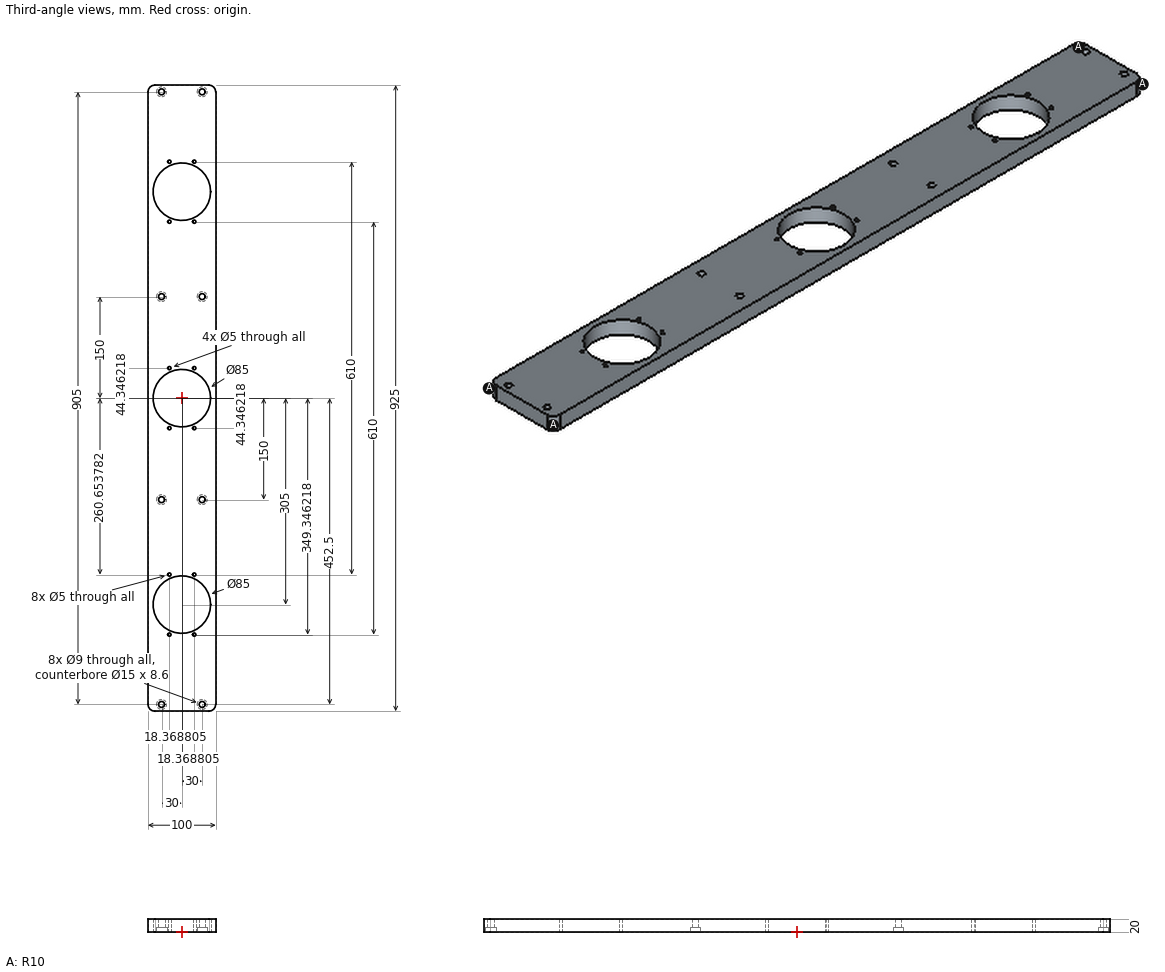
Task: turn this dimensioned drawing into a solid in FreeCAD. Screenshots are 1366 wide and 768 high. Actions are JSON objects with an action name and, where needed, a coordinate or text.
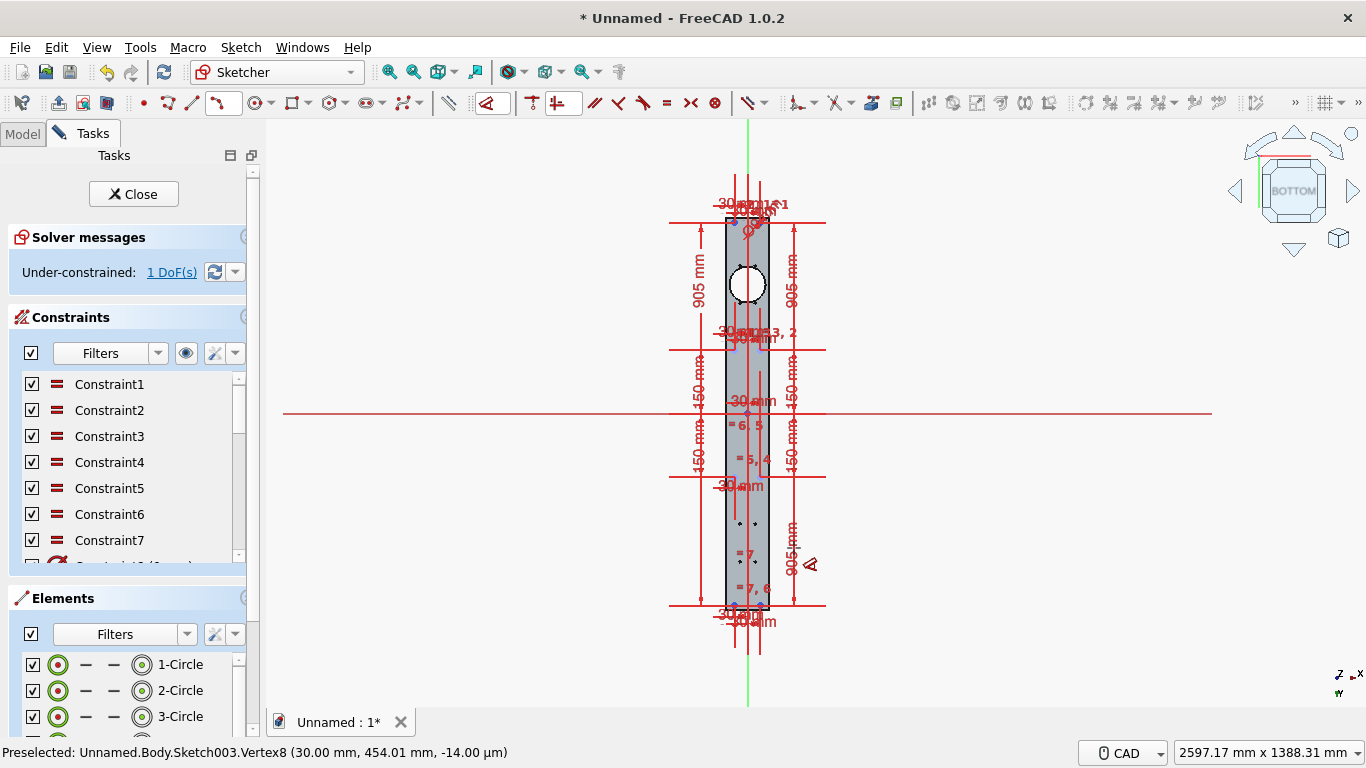
{"action": "left_click", "coordinate": [760, 223]}
{"action": "left_click", "coordinate": [794, 362]}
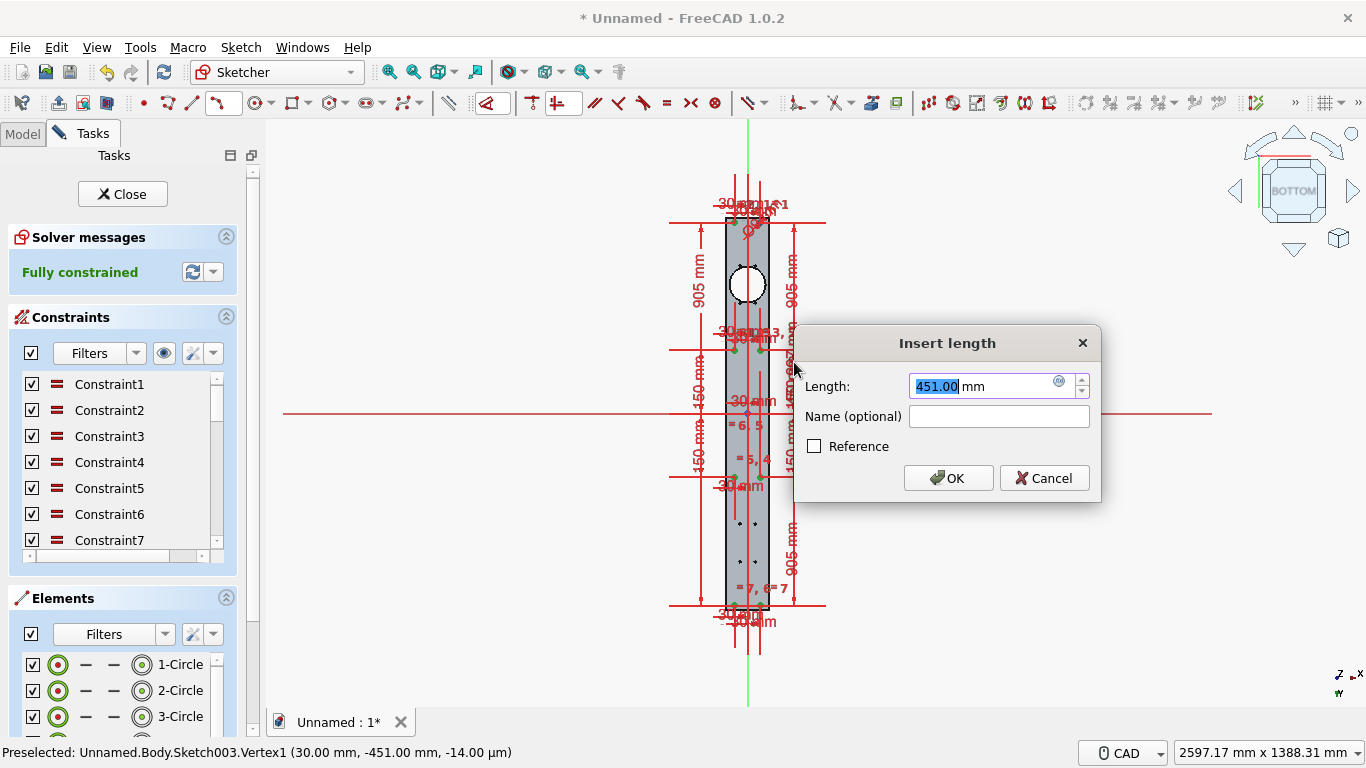
{"action": "type", "text": "452.5"}
{"action": "key", "text": "Return"}
{"action": "key", "text": "Escape"}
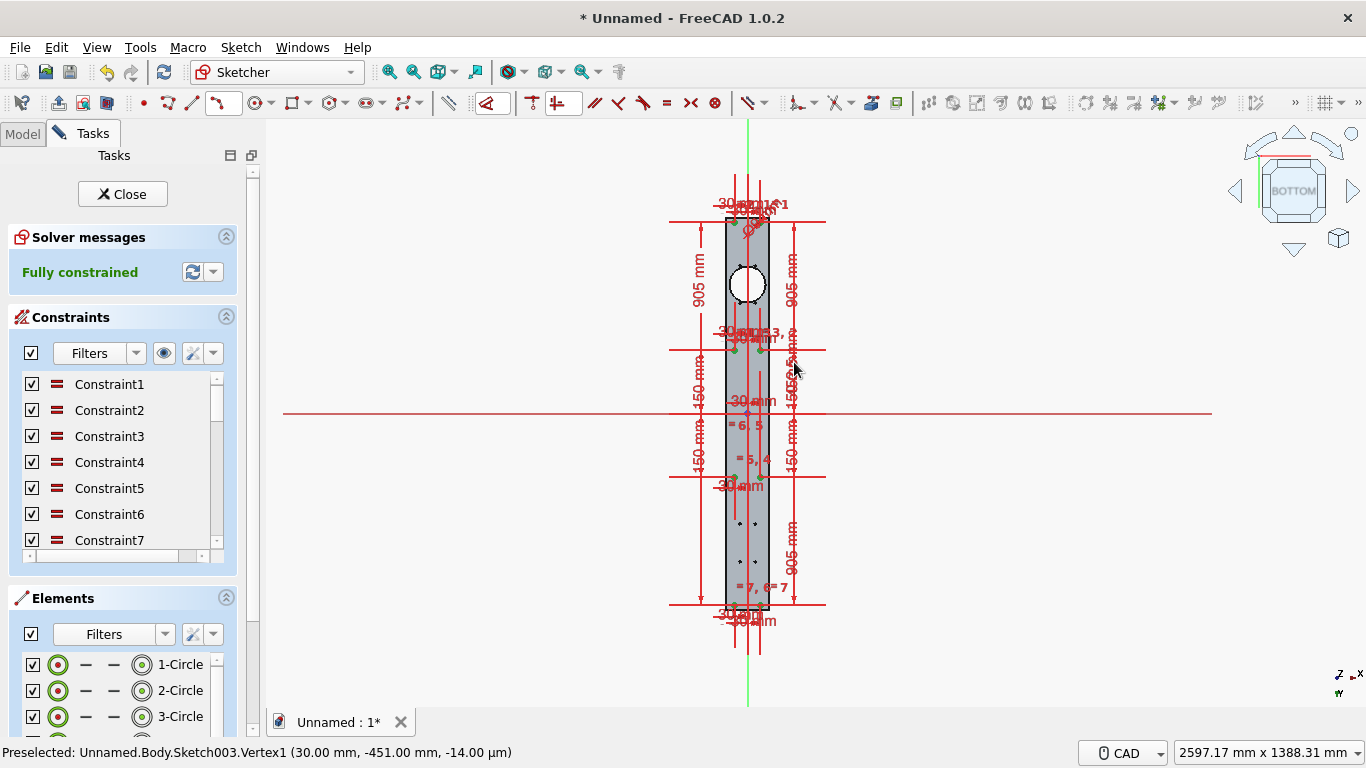
{"action": "left_click", "coordinate": [123, 194]}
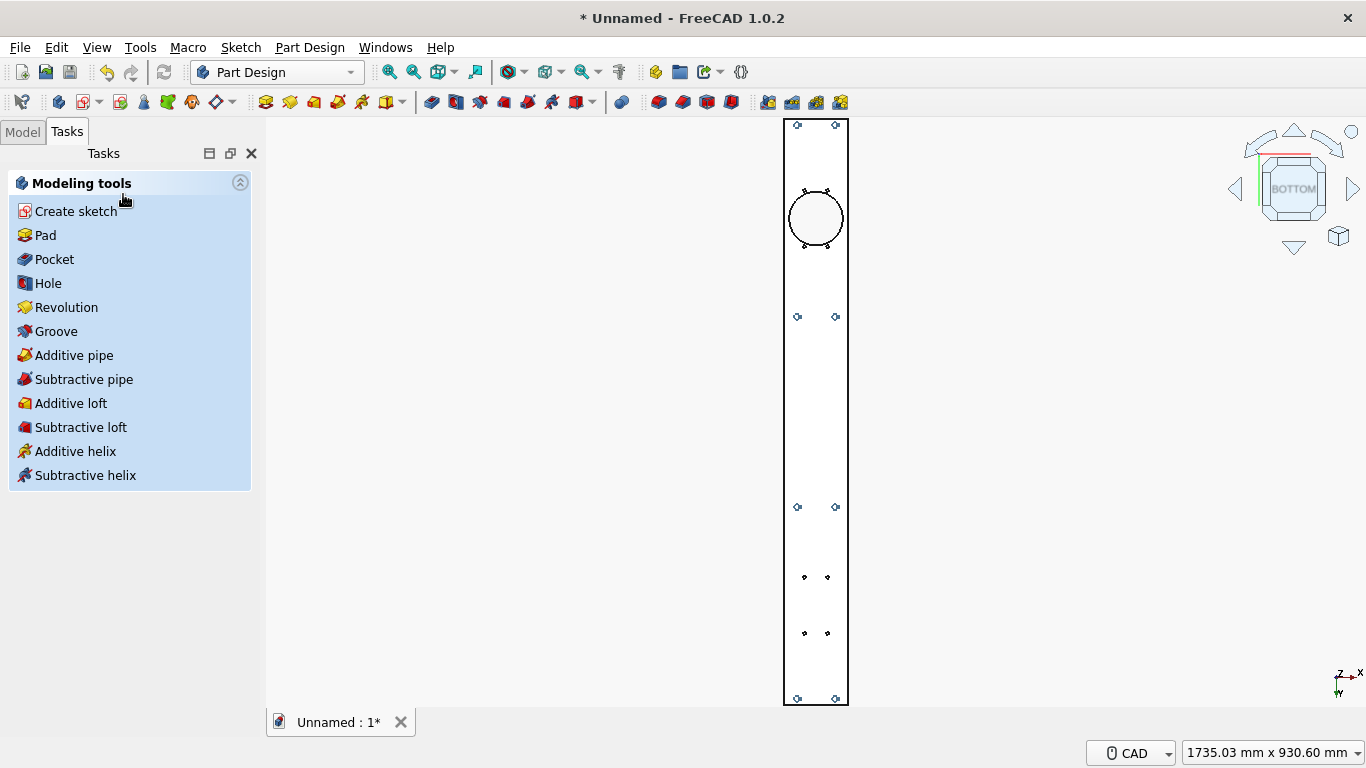
{"action": "left_click", "coordinate": [456, 102]}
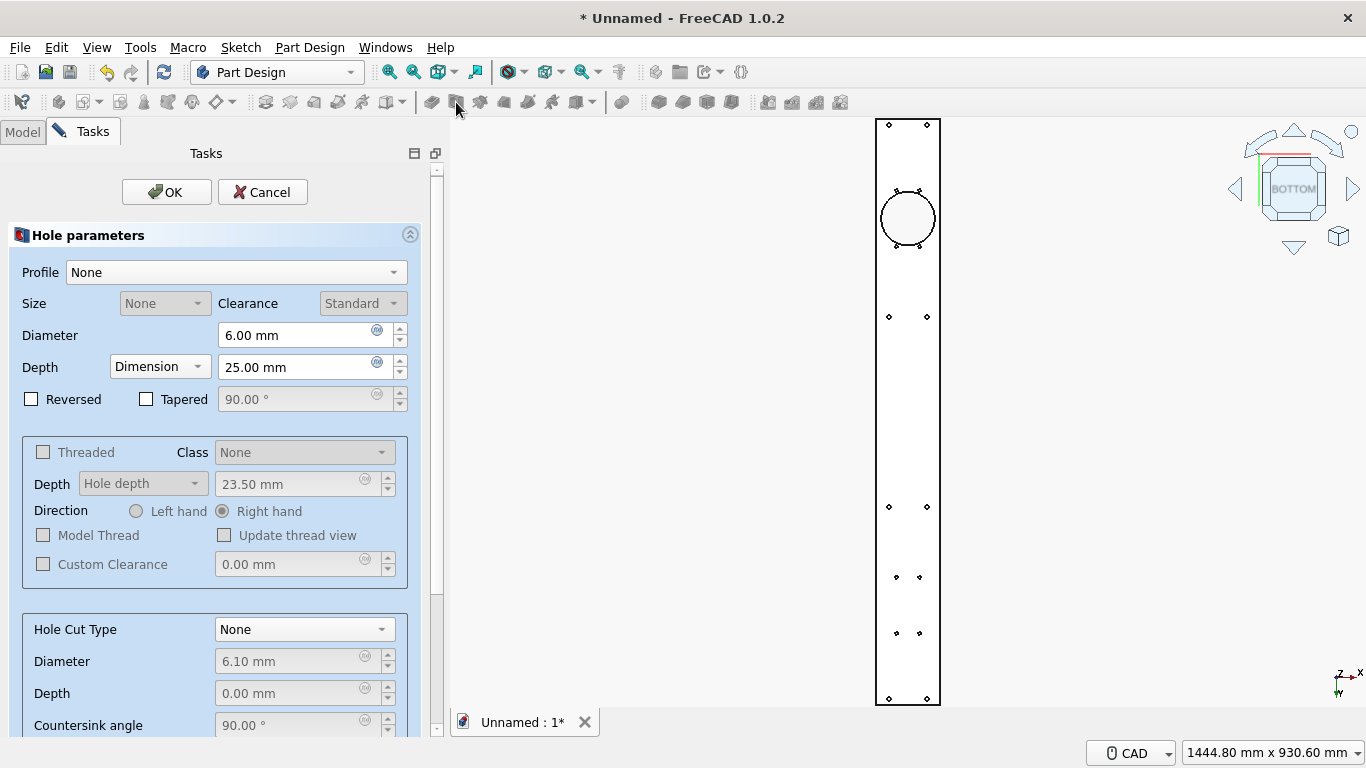
{"action": "triple_click", "coordinate": [305, 335]}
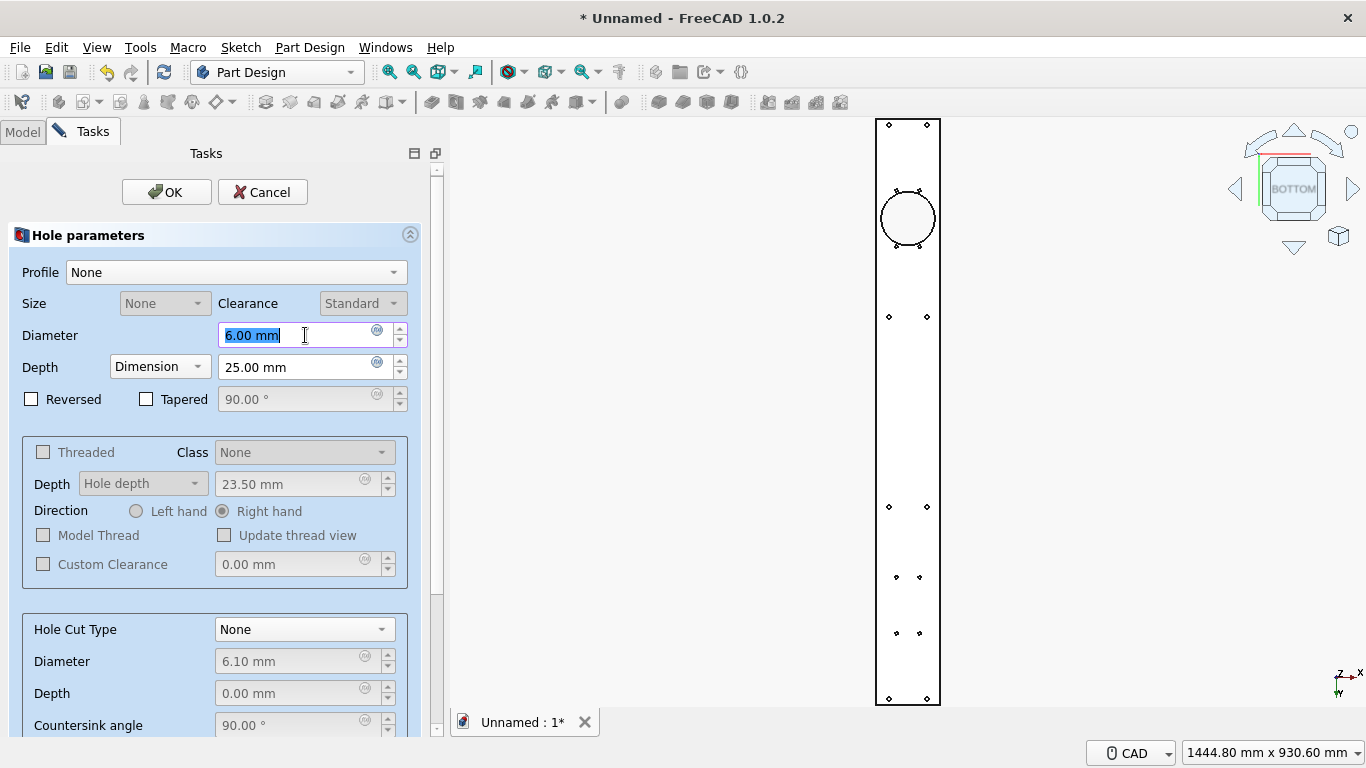
{"action": "type", "text": "9"}
{"action": "key", "text": "Tab"}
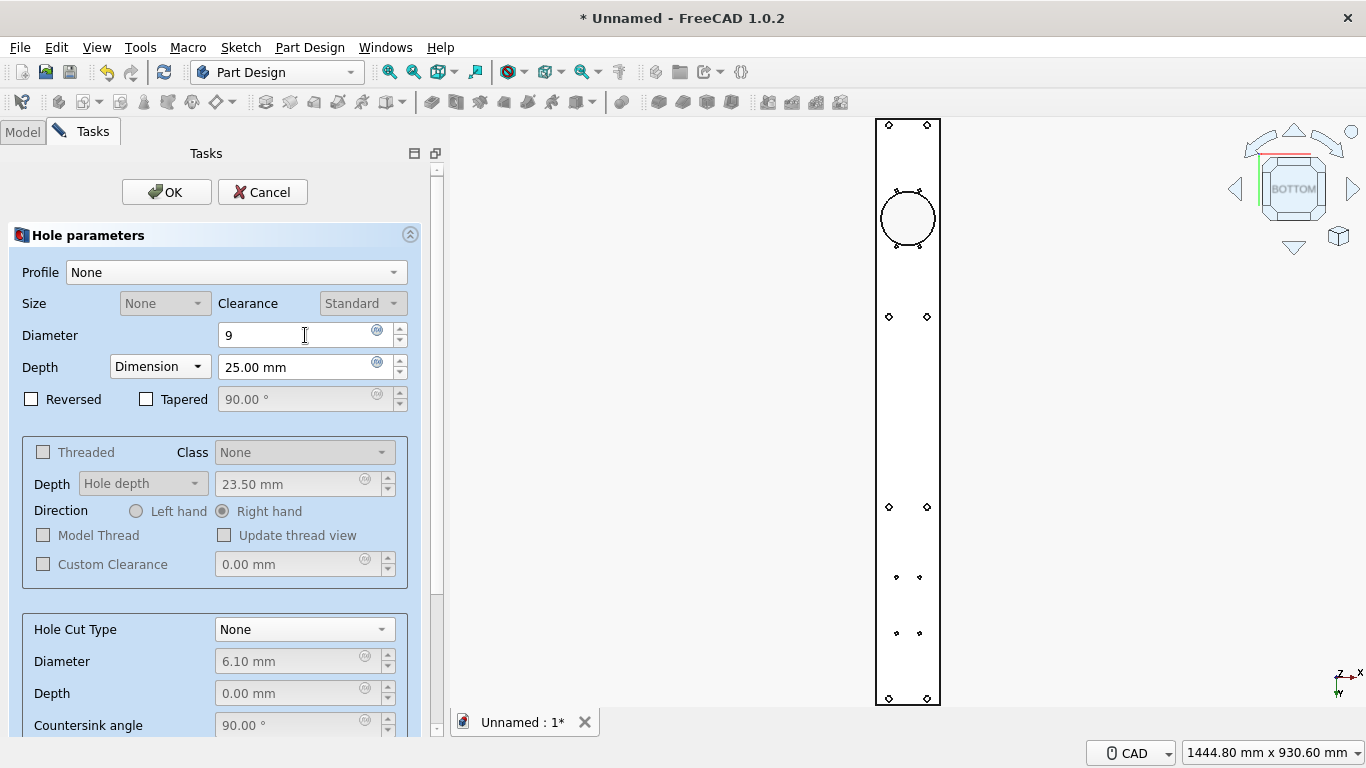
{"action": "left_click", "coordinate": [161, 366]}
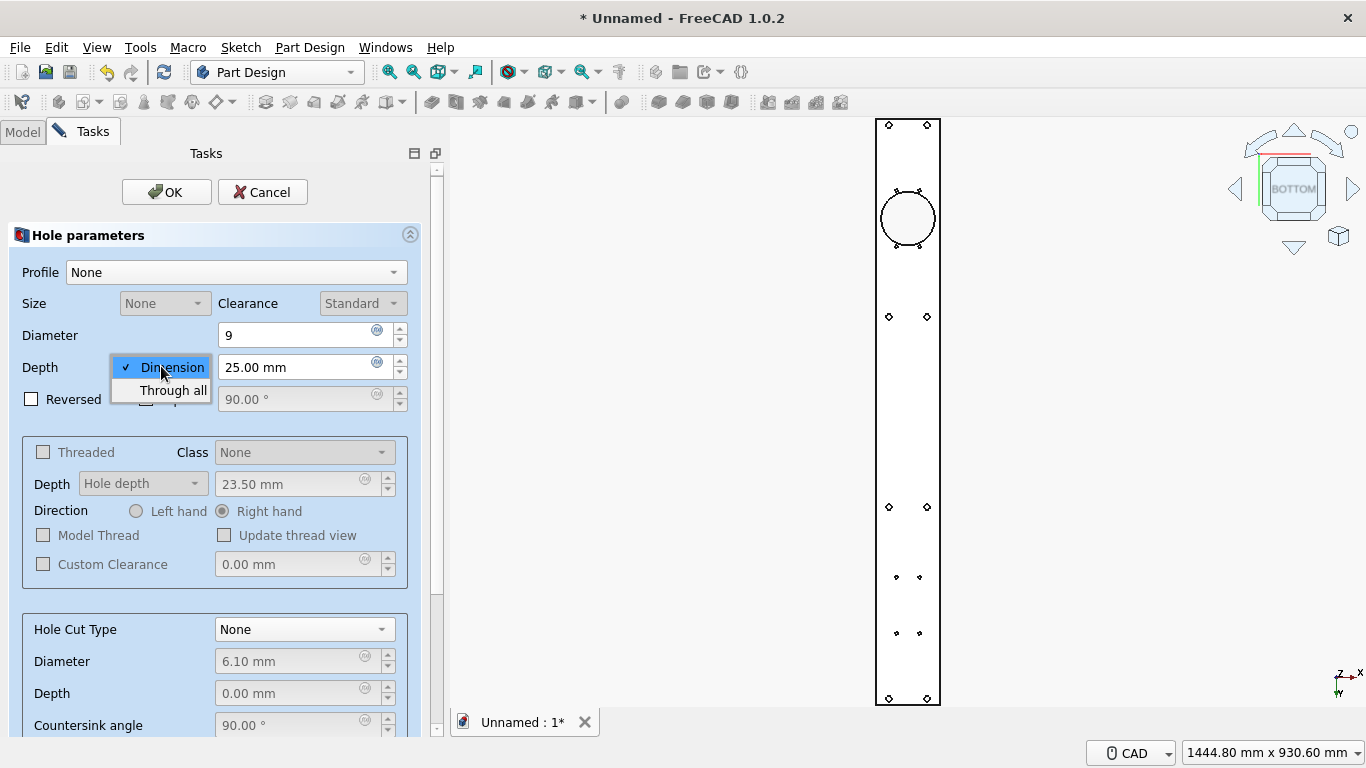
{"action": "left_click", "coordinate": [160, 390]}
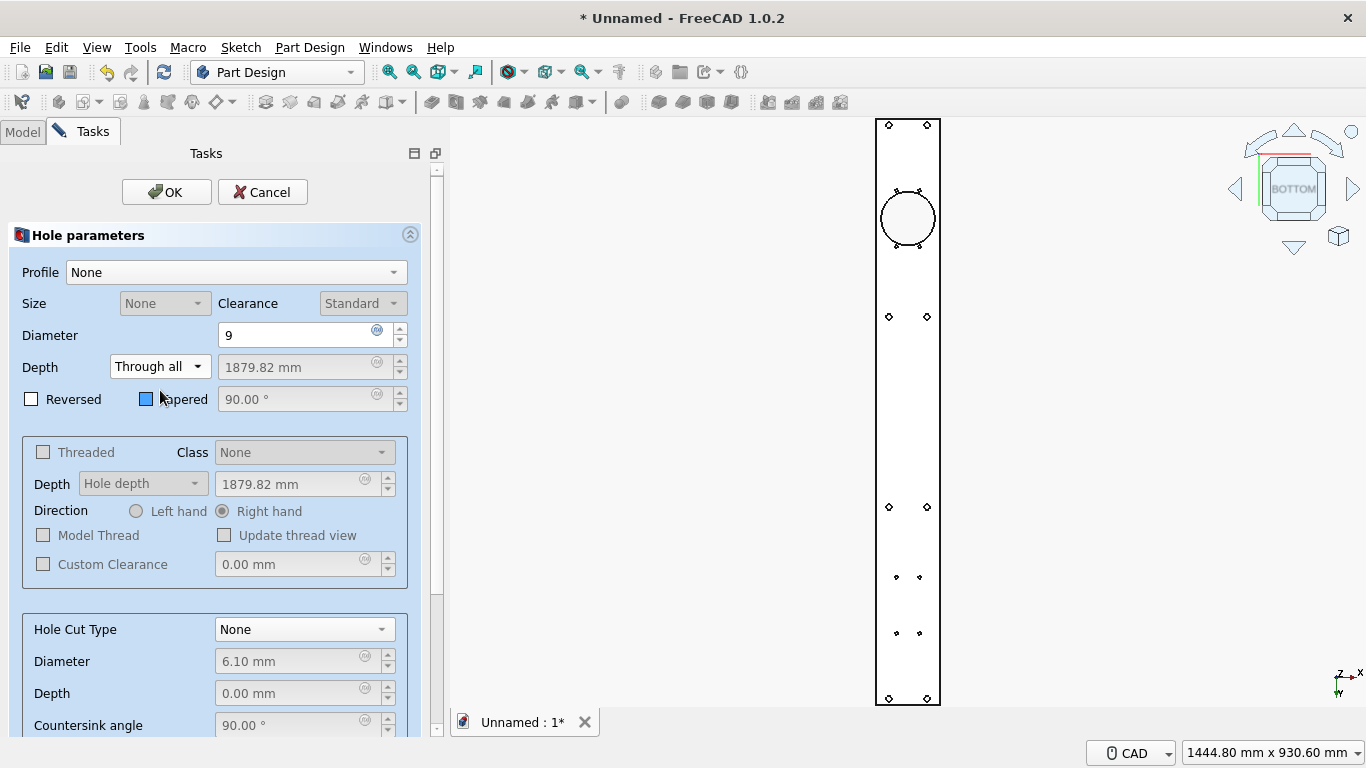
{"action": "left_click", "coordinate": [306, 630]}